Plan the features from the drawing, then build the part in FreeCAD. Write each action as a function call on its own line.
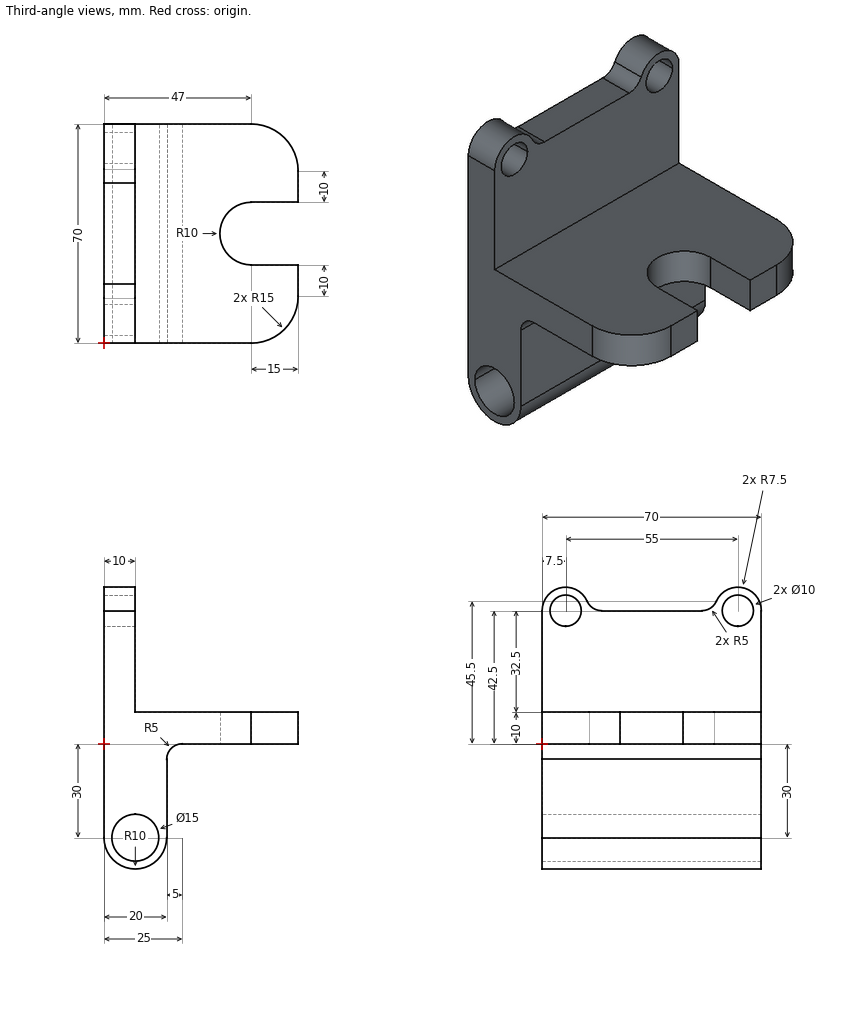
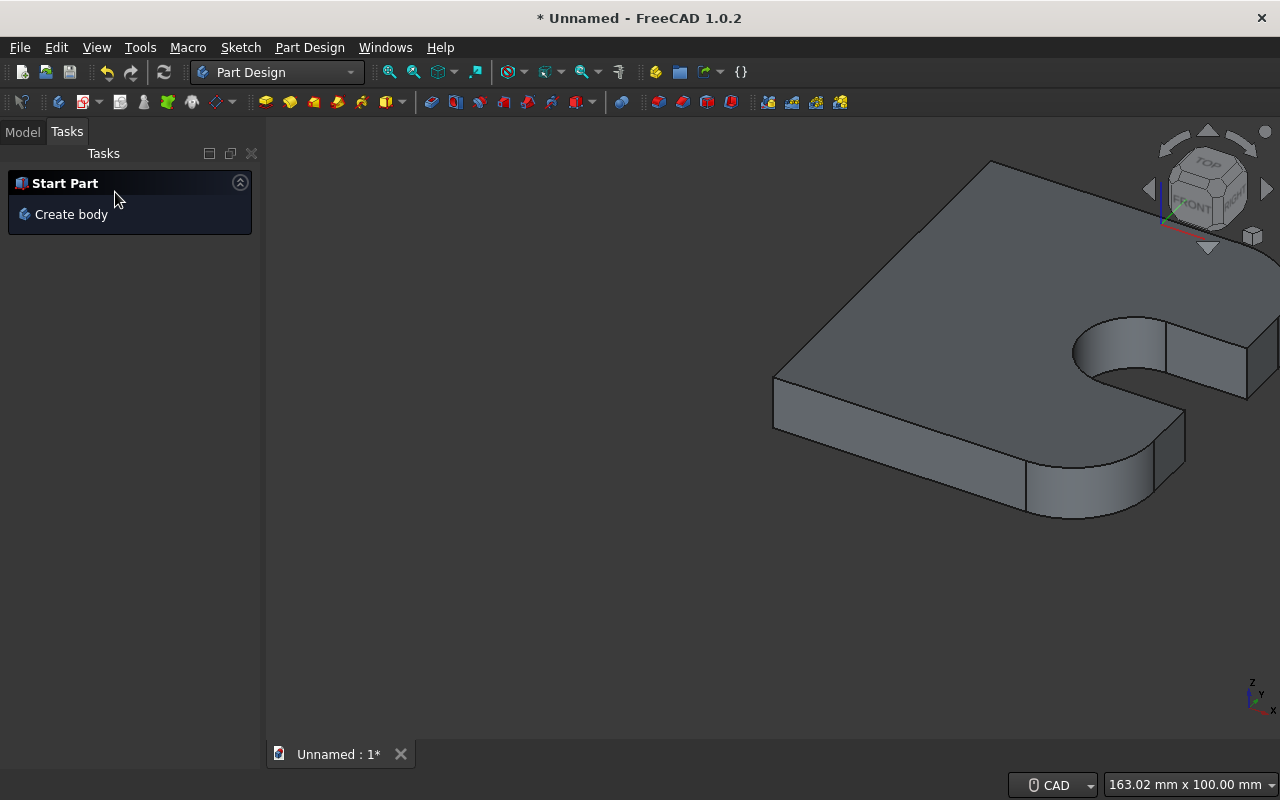
click(390, 72)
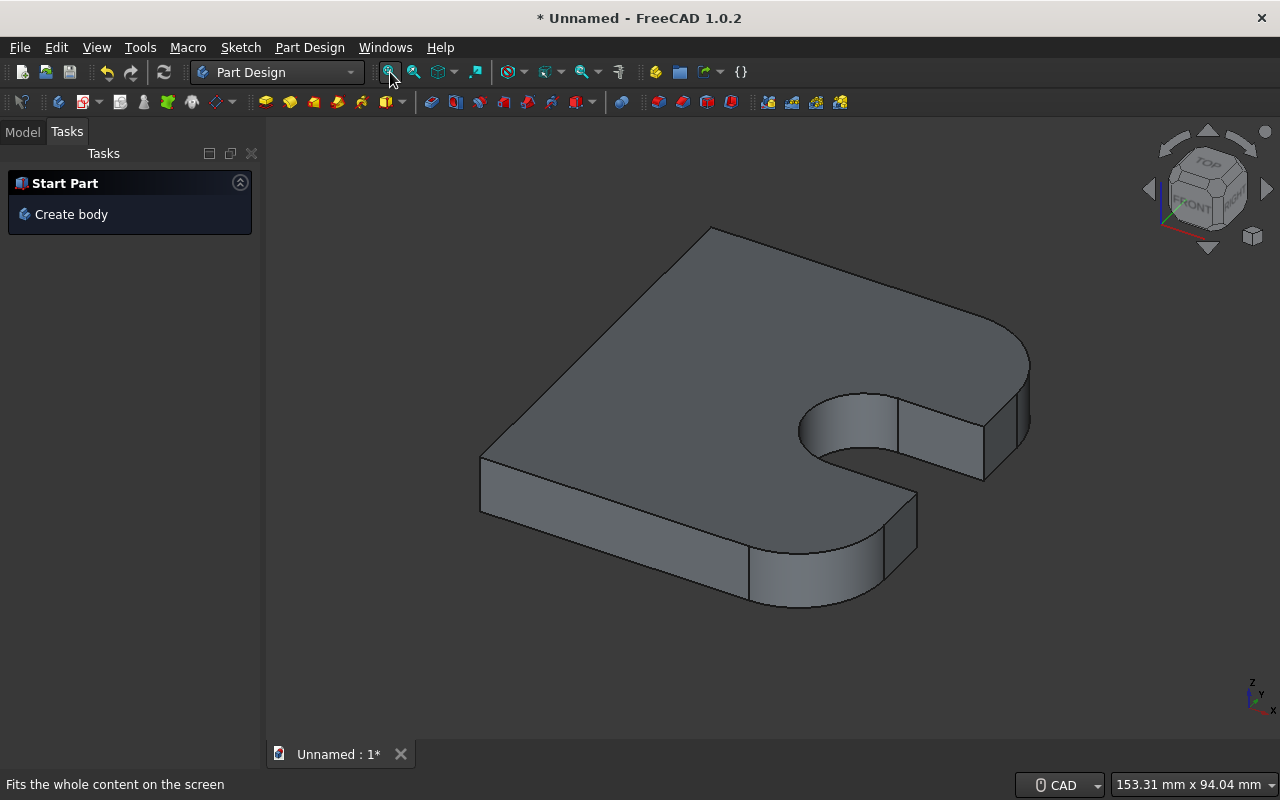
click(84, 102)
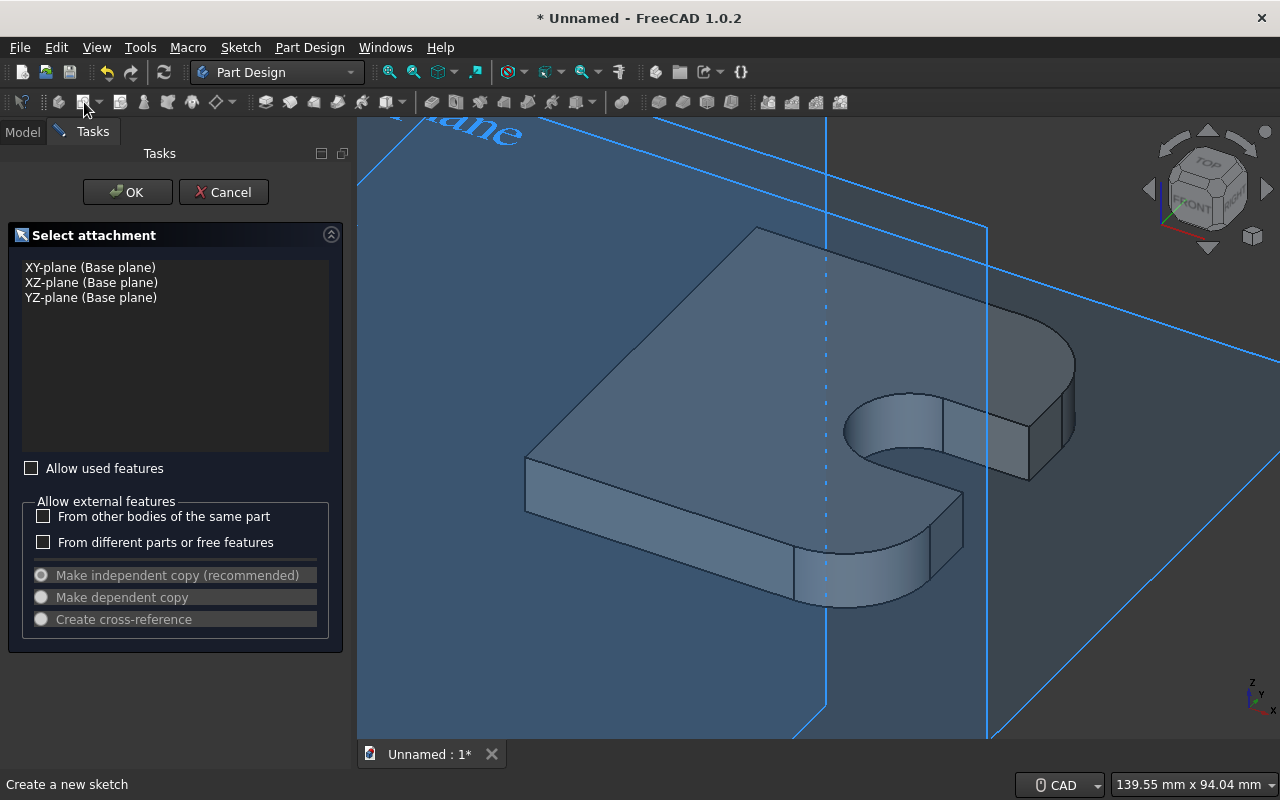
click(82, 298)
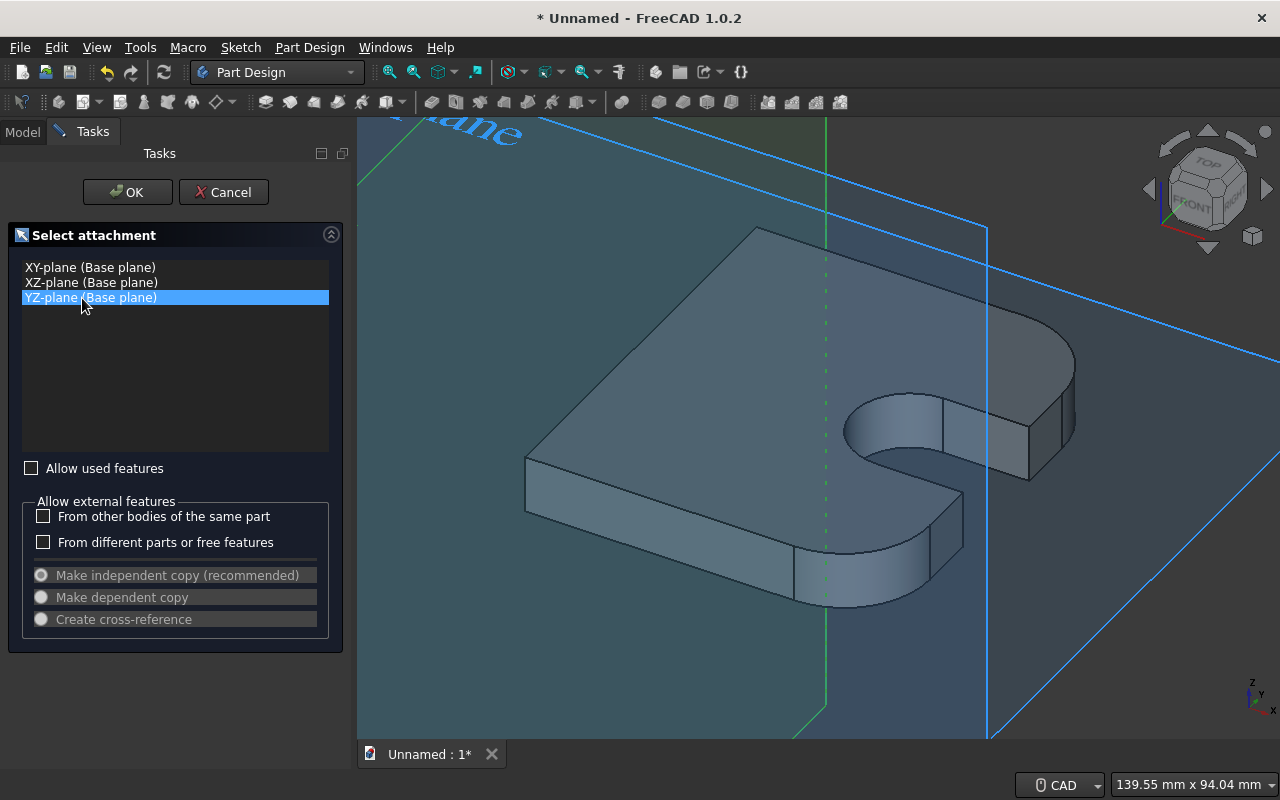
click(128, 192)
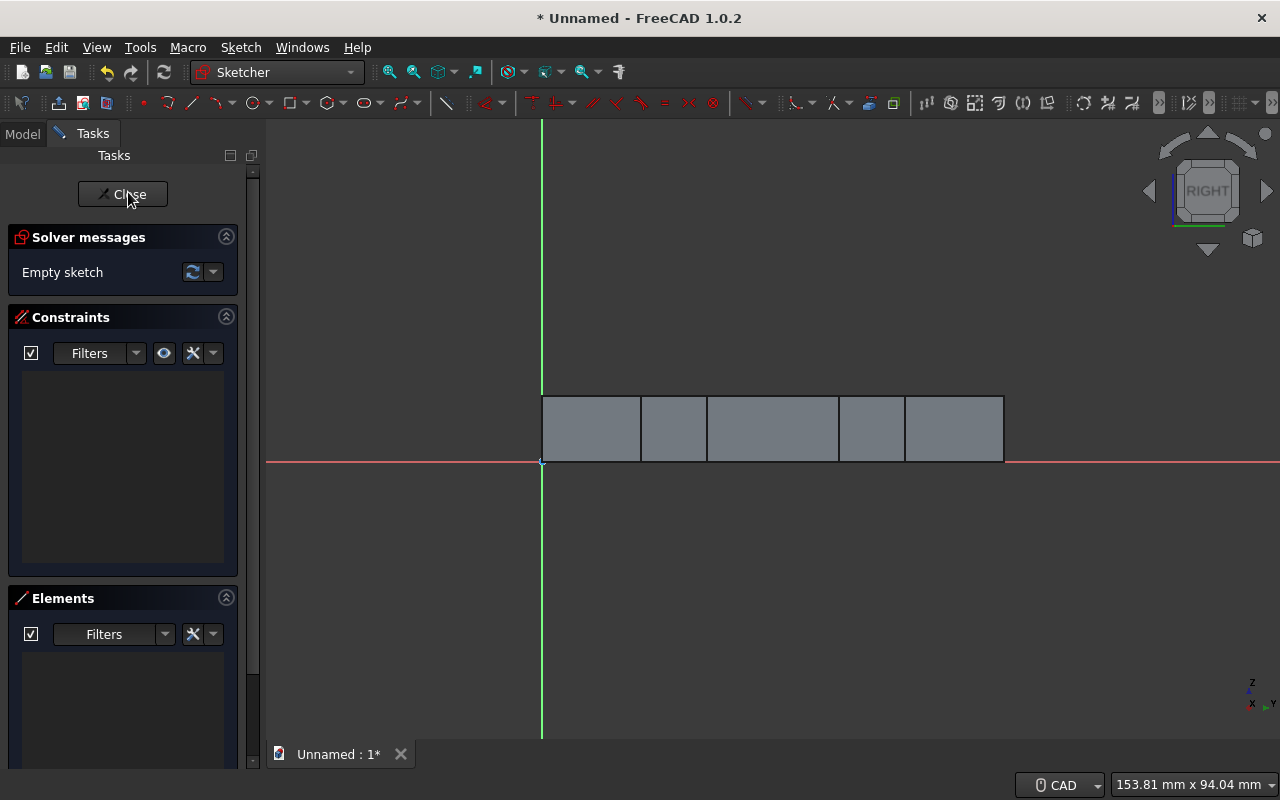
click(108, 104)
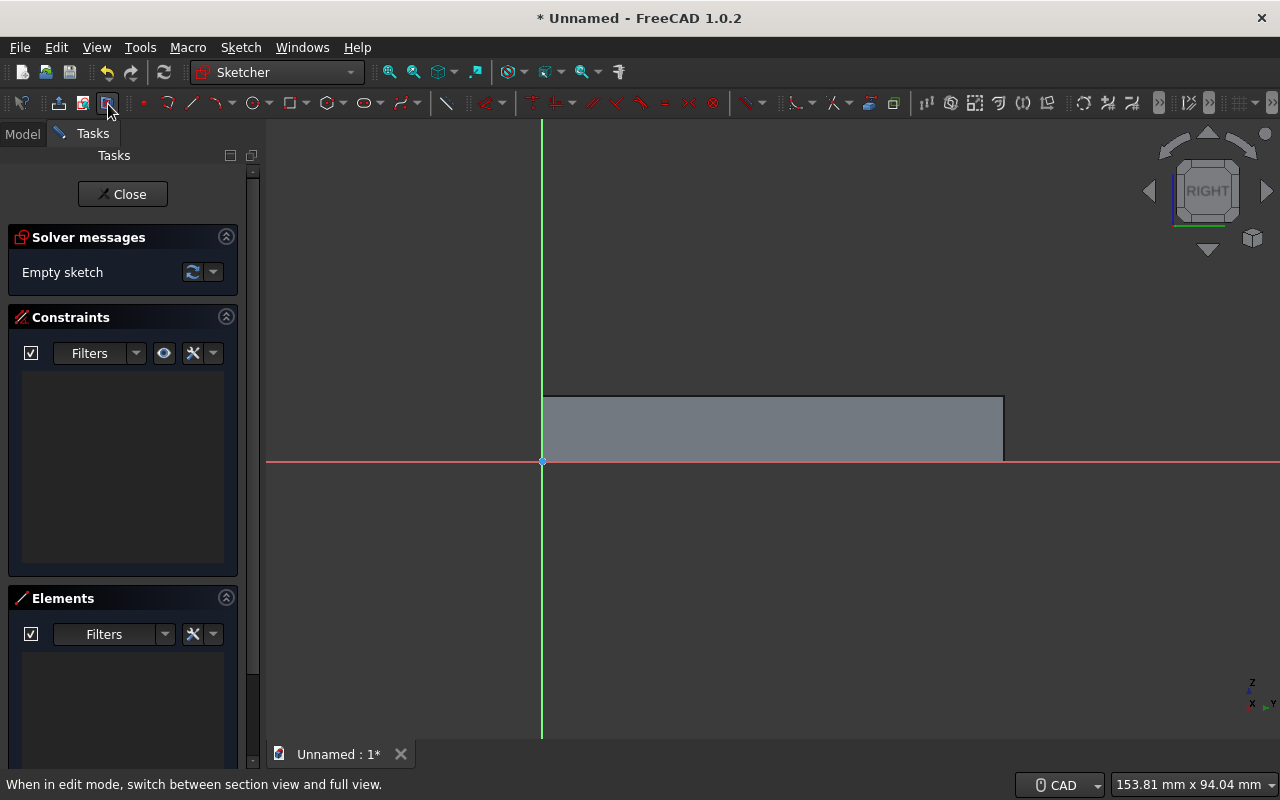
click(290, 104)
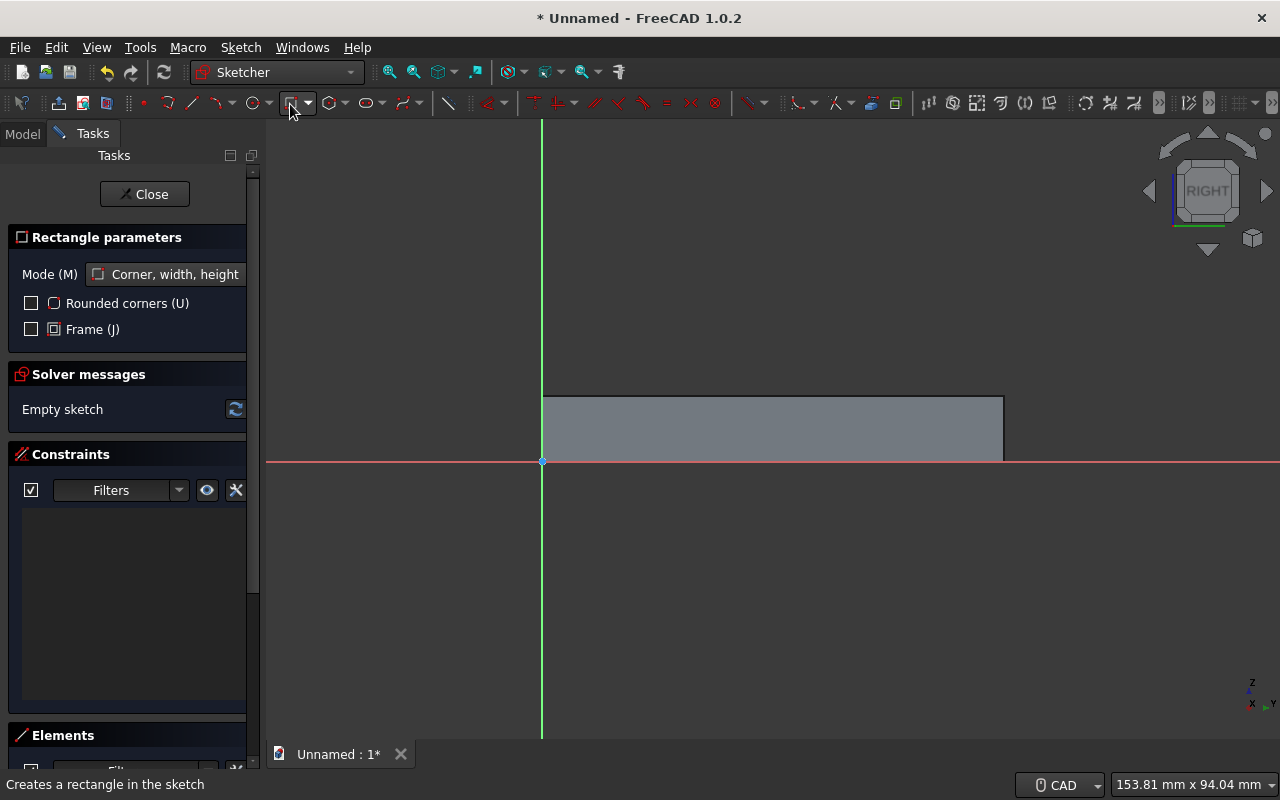
click(542, 182)
click(1004, 396)
key(Escape)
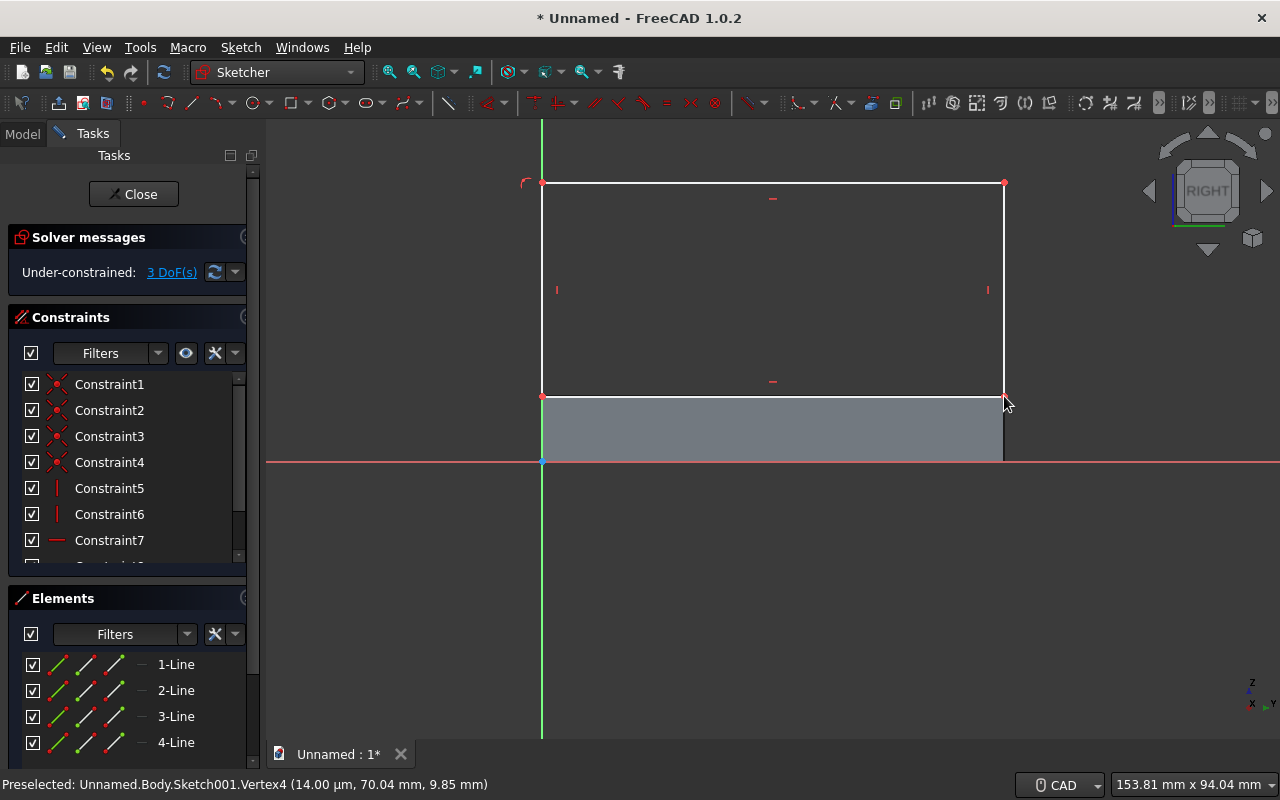
click(488, 104)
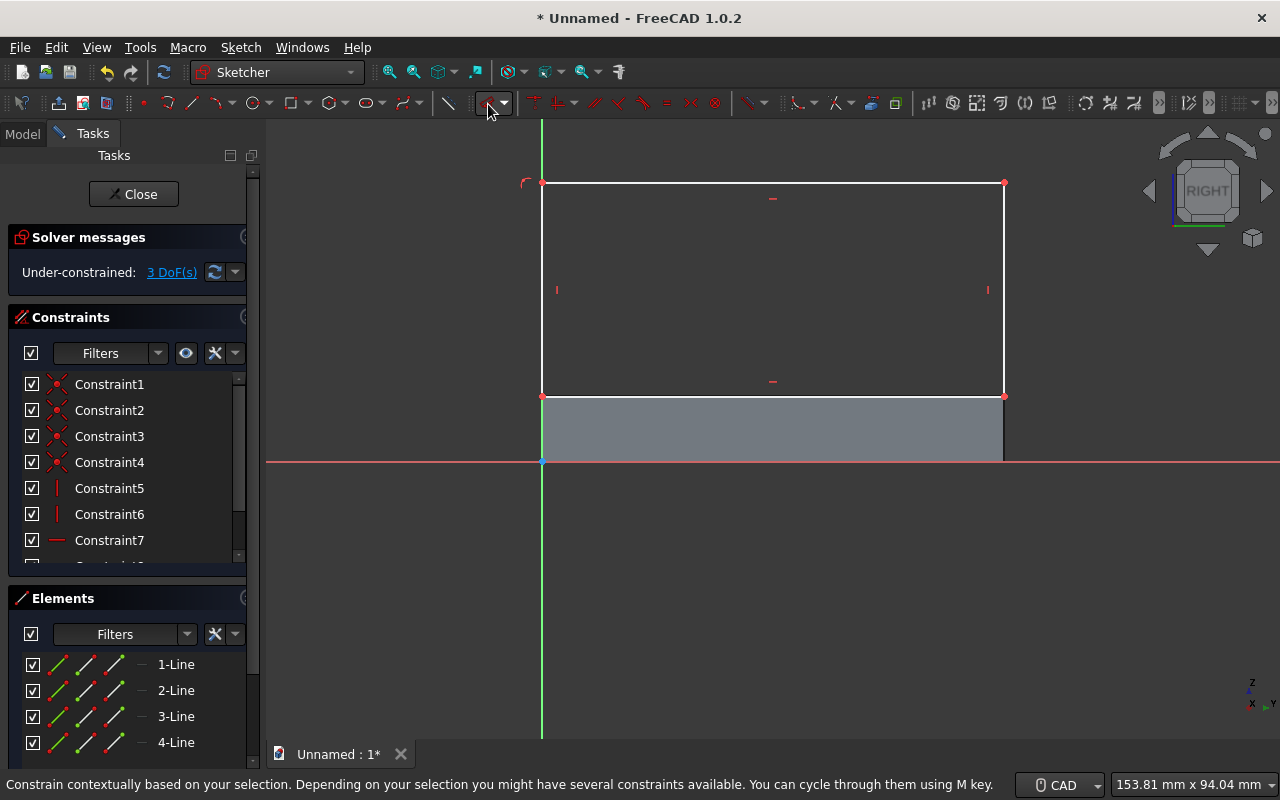
click(681, 397)
click(773, 431)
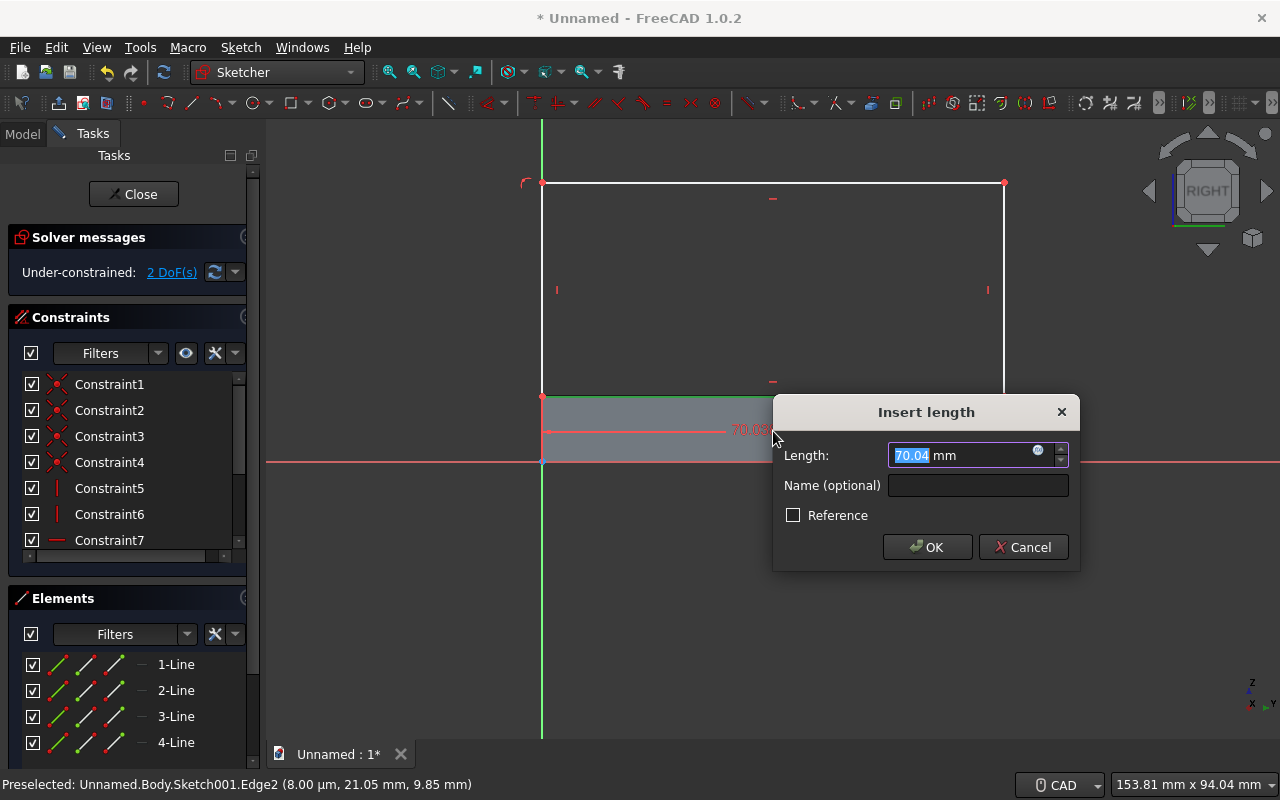
text(70)
key(Return)